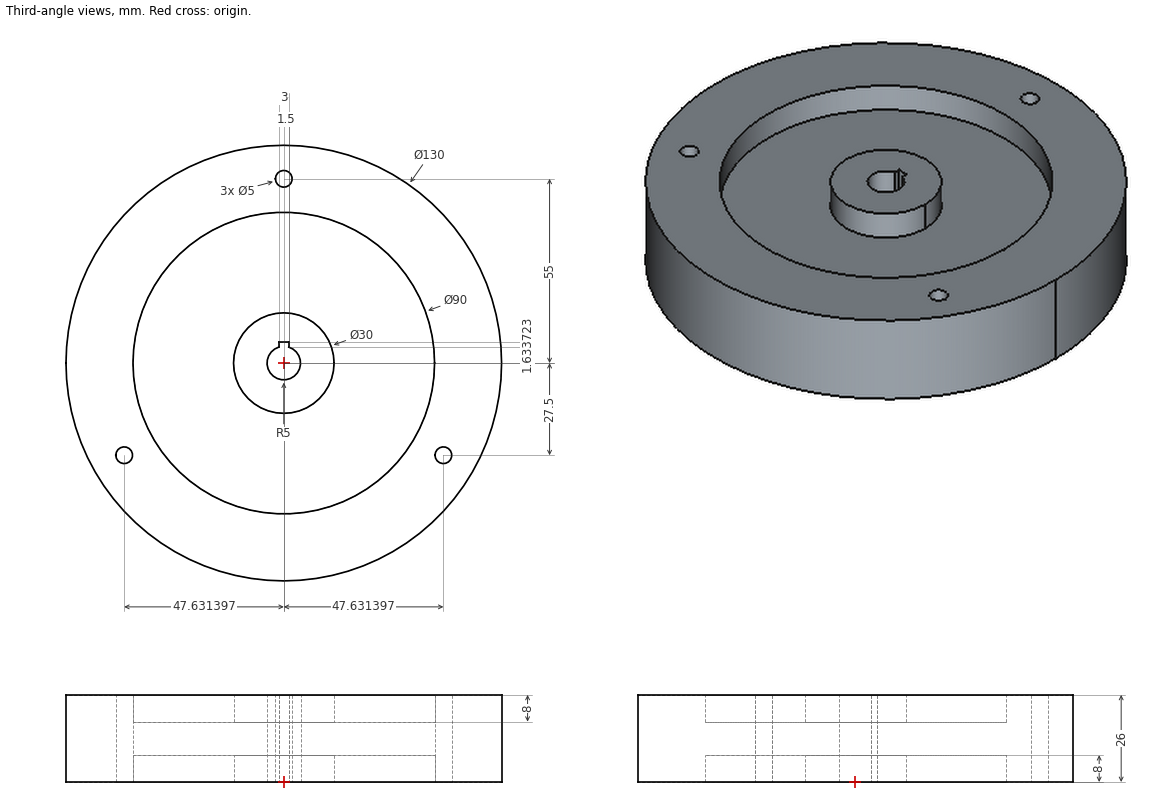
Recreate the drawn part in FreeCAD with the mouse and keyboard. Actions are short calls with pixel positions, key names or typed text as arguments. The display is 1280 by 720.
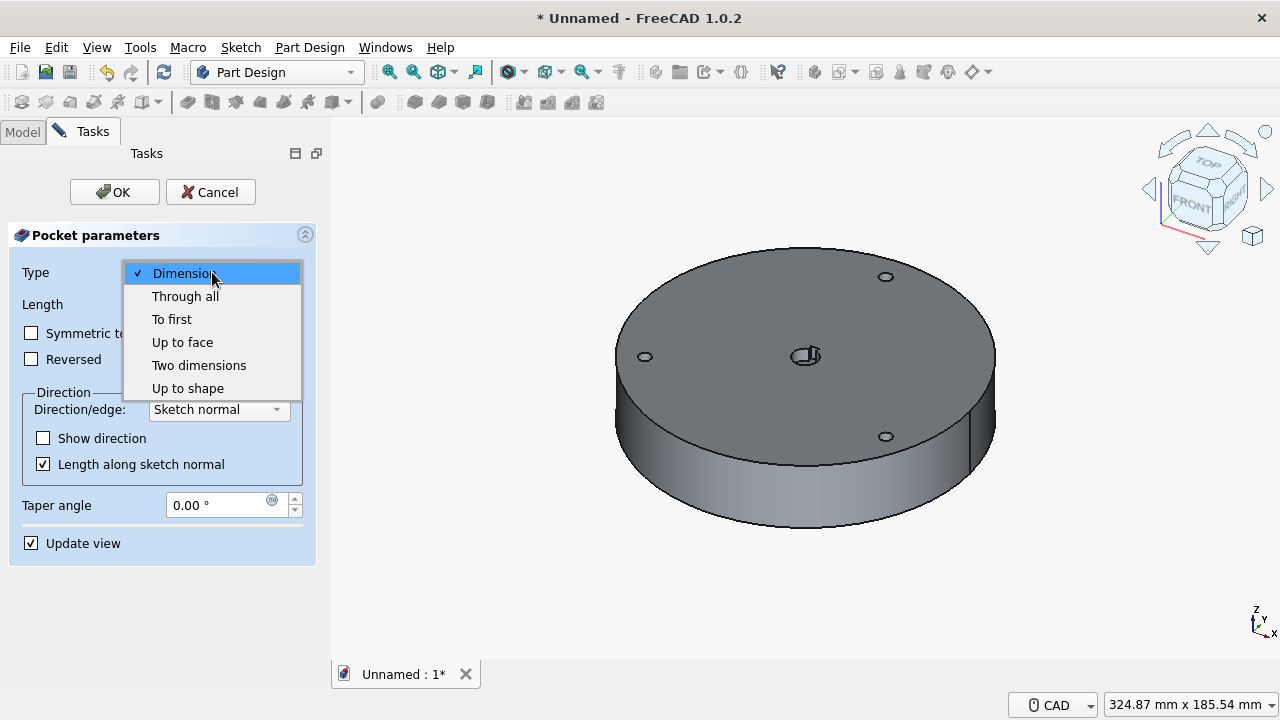
click(212, 296)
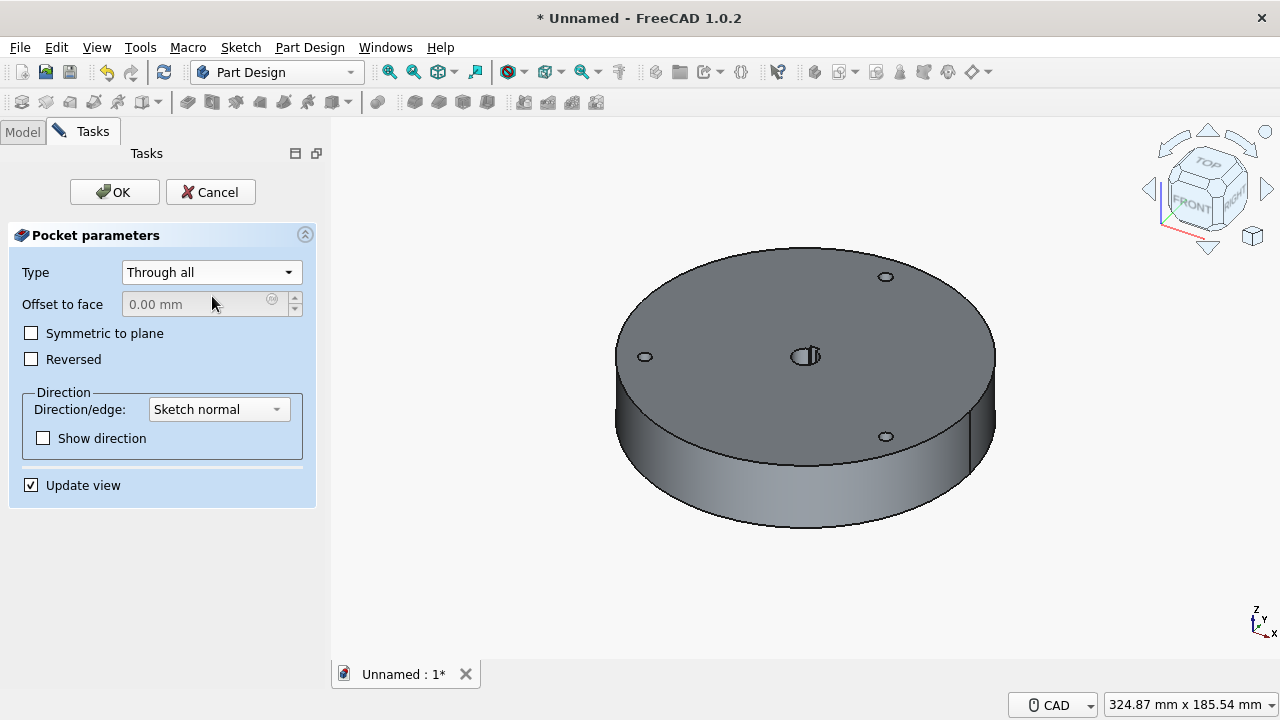
click(115, 192)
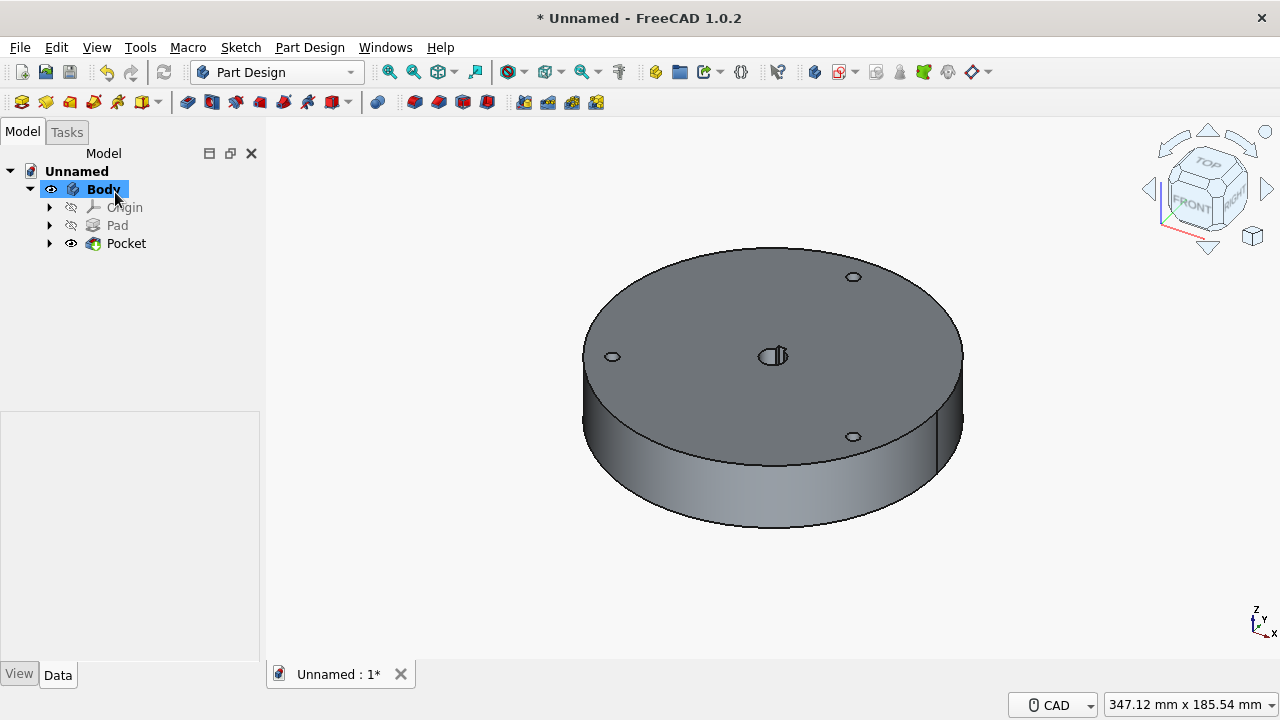
click(719, 410)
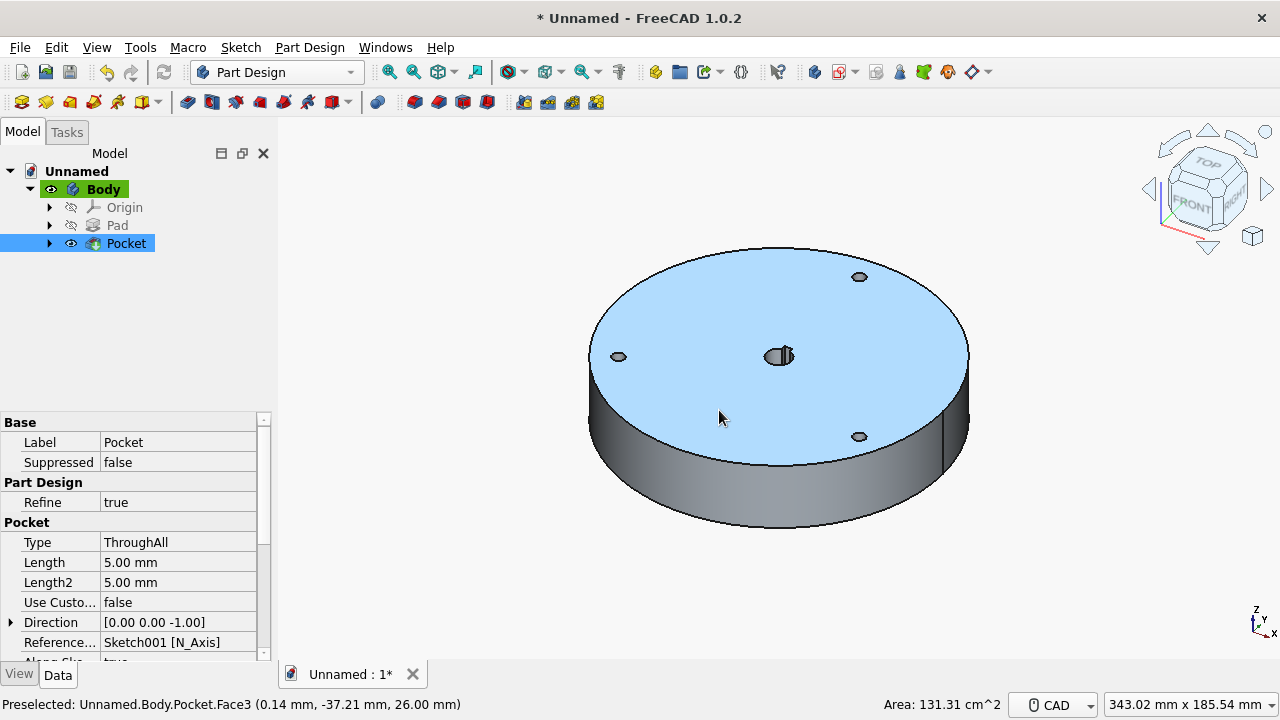
click(840, 72)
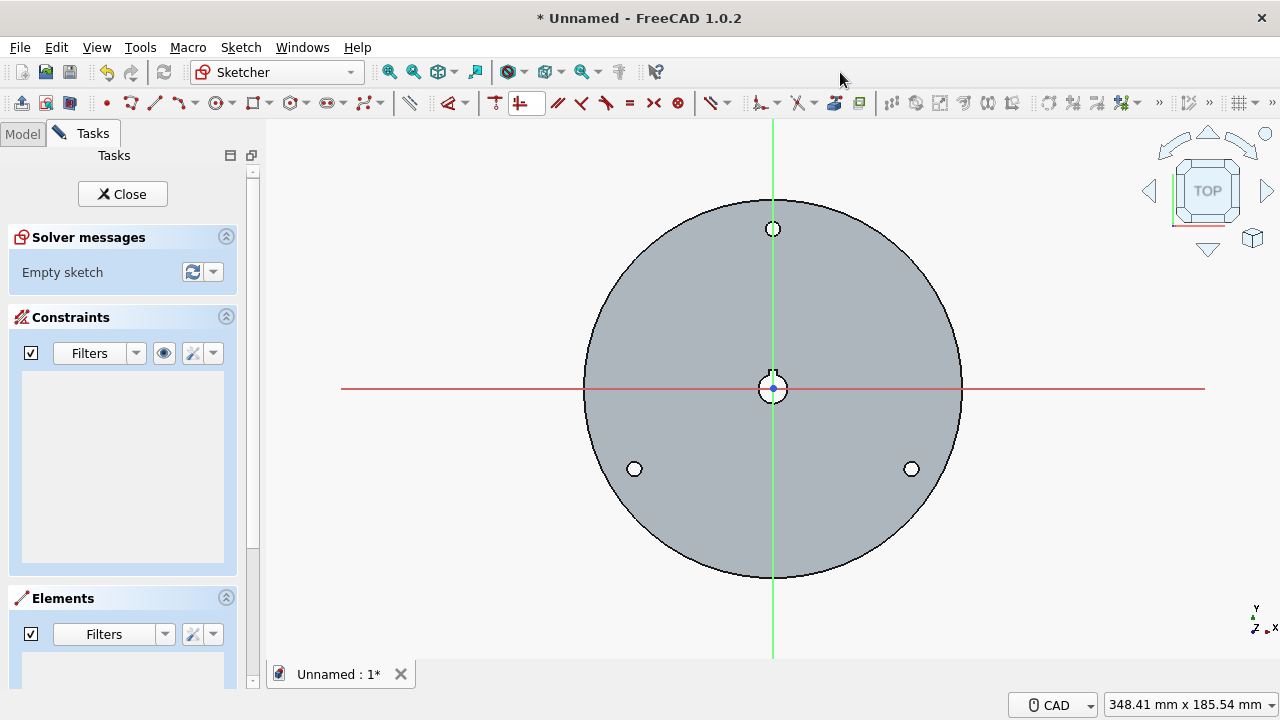
click(216, 104)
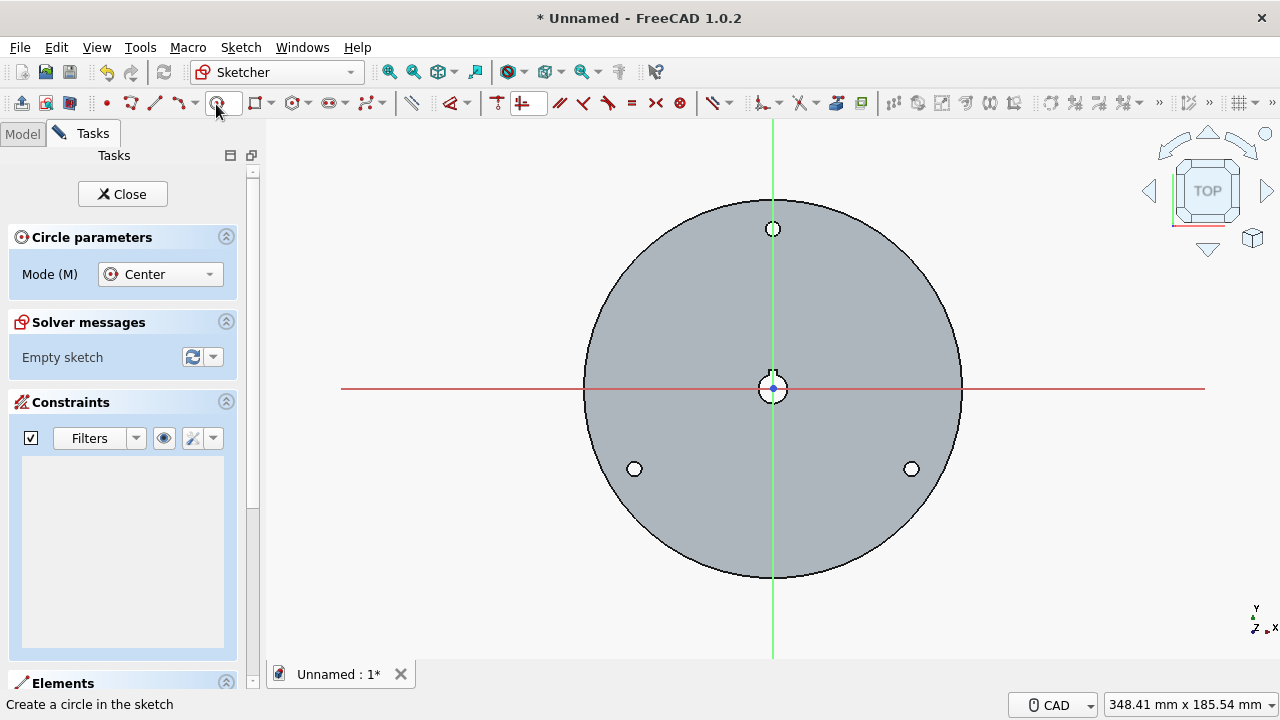
click(773, 389)
click(866, 296)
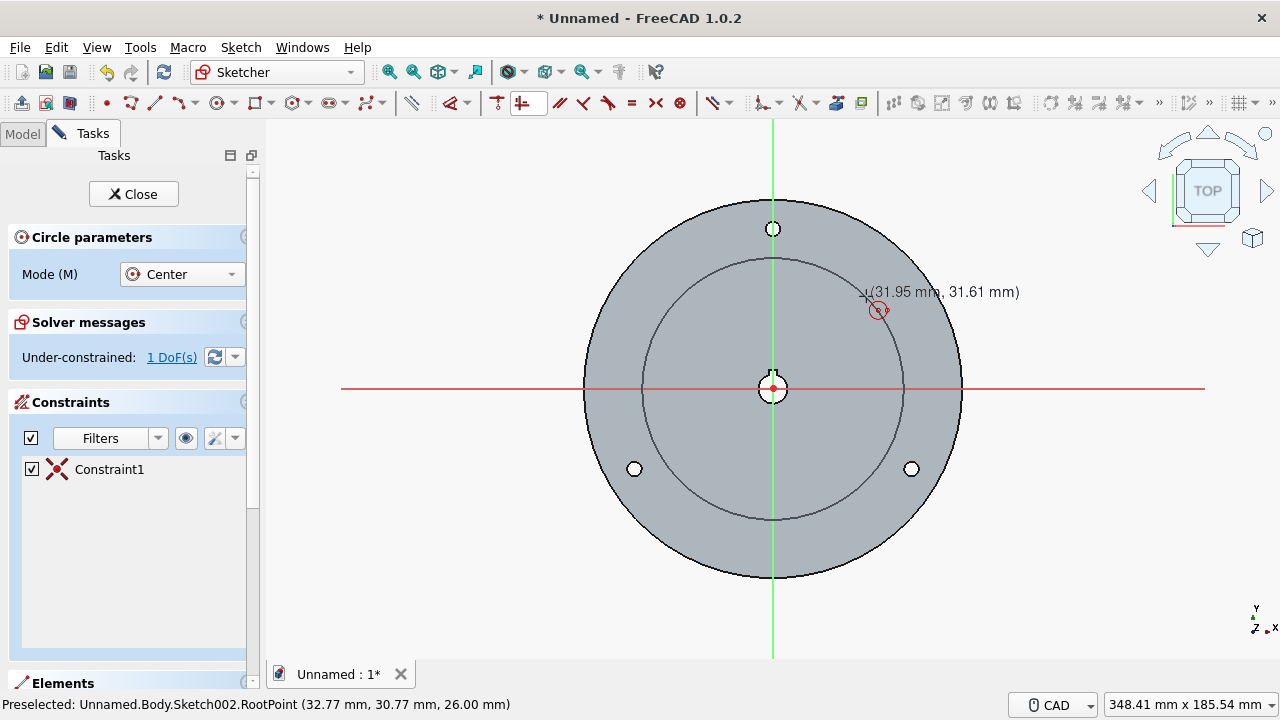
click(773, 389)
click(804, 358)
key(Escape)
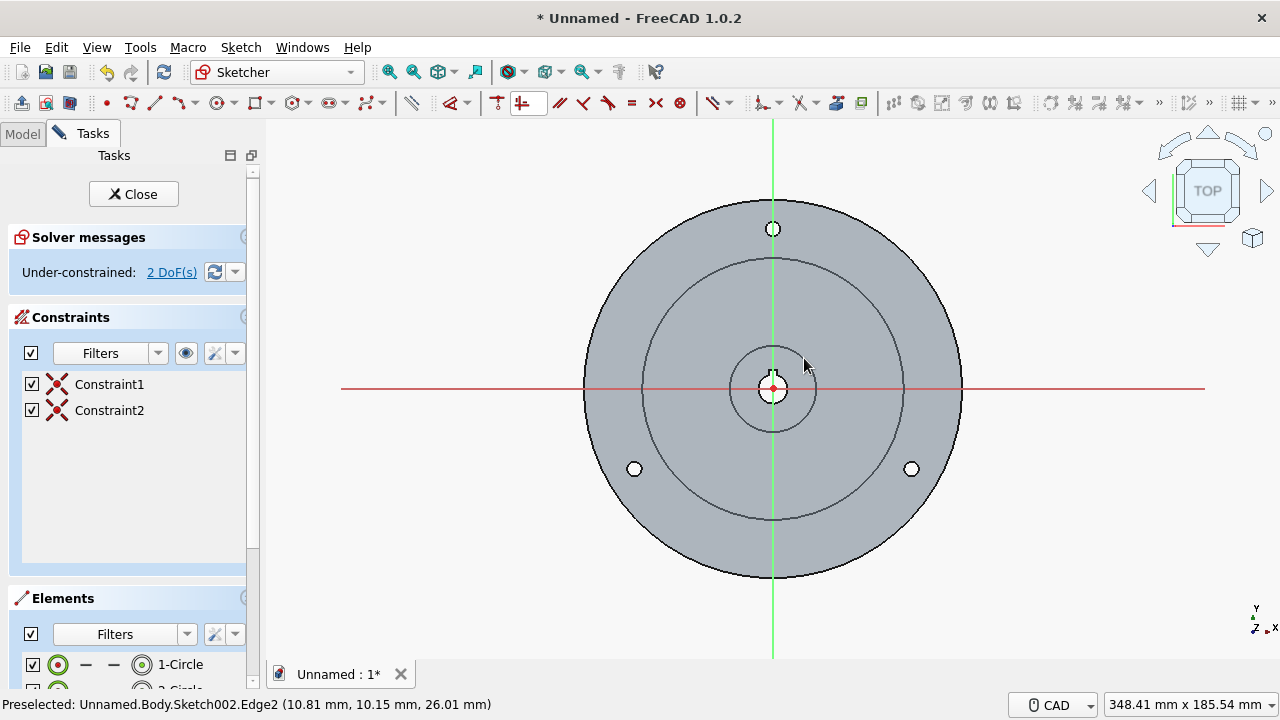
key(d)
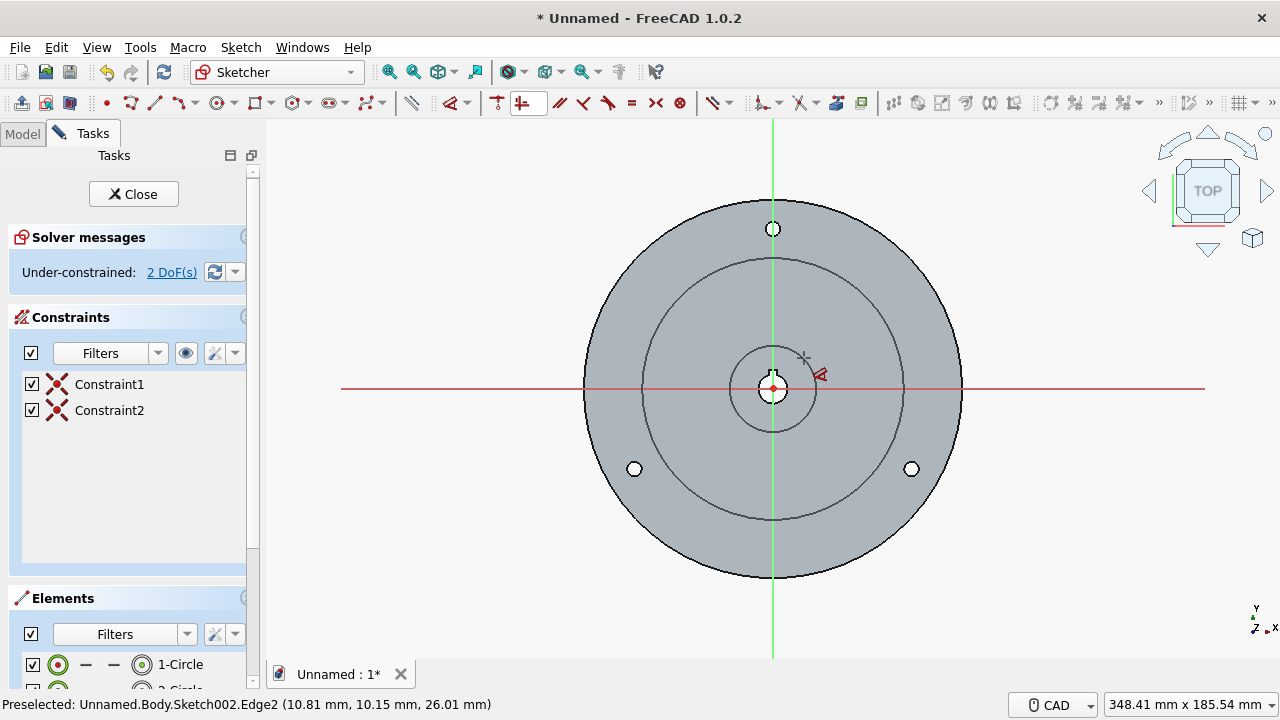
click(865, 296)
click(888, 273)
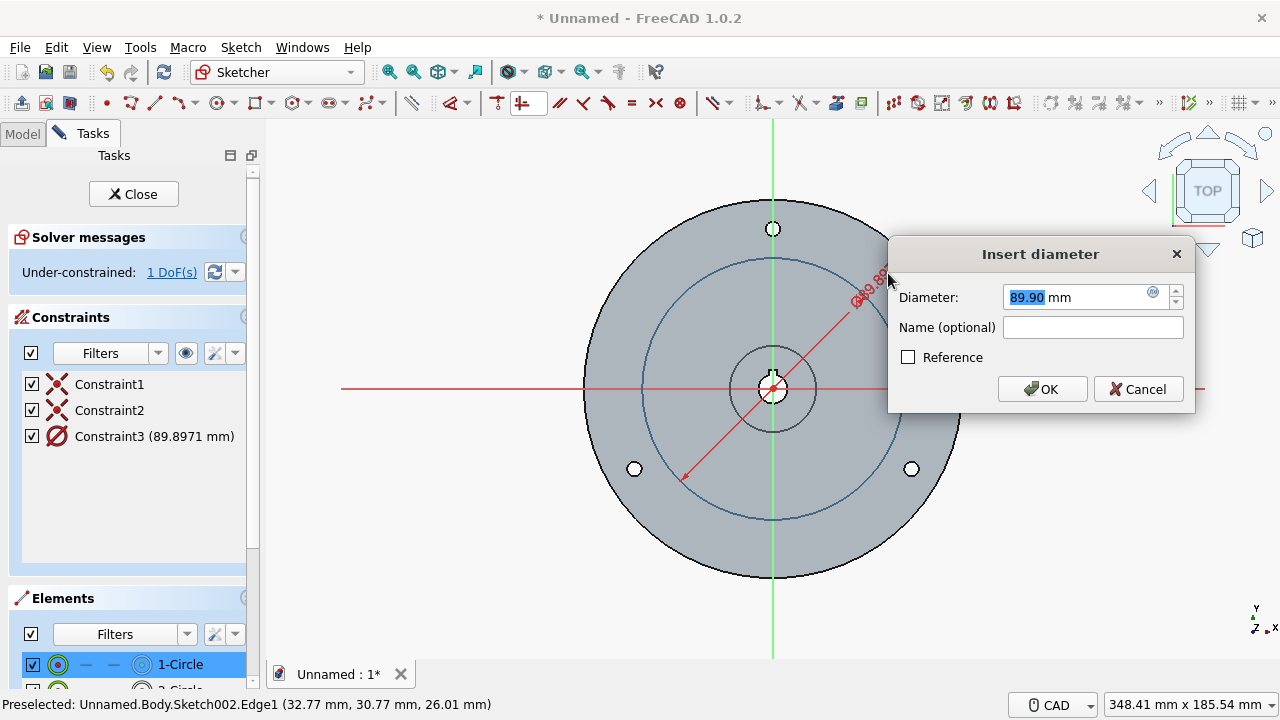
text(90)
key(Return)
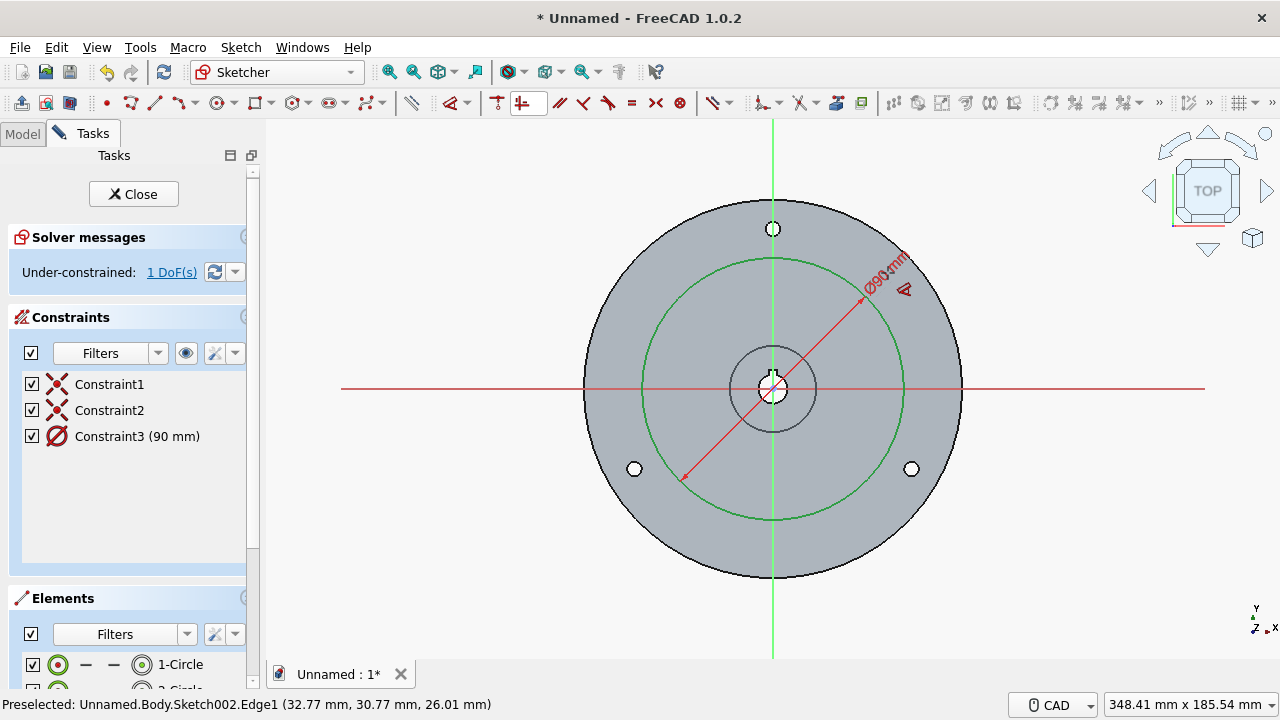
click(803, 358)
click(825, 335)